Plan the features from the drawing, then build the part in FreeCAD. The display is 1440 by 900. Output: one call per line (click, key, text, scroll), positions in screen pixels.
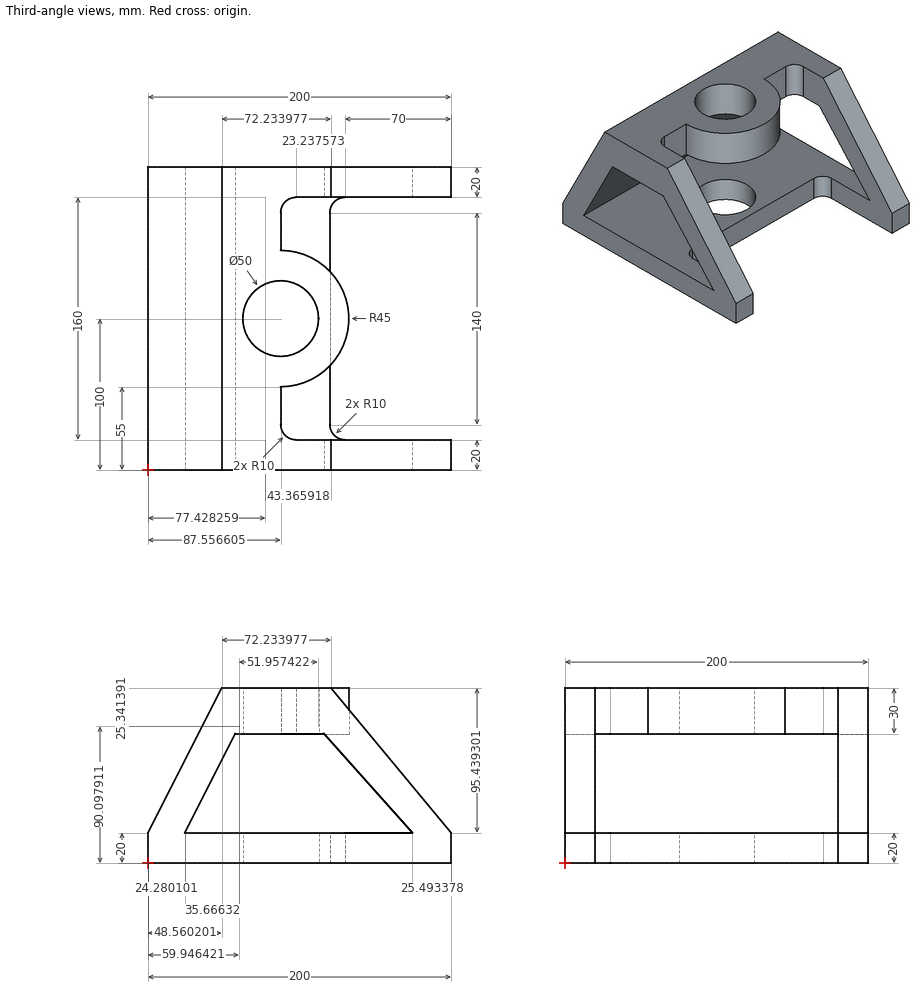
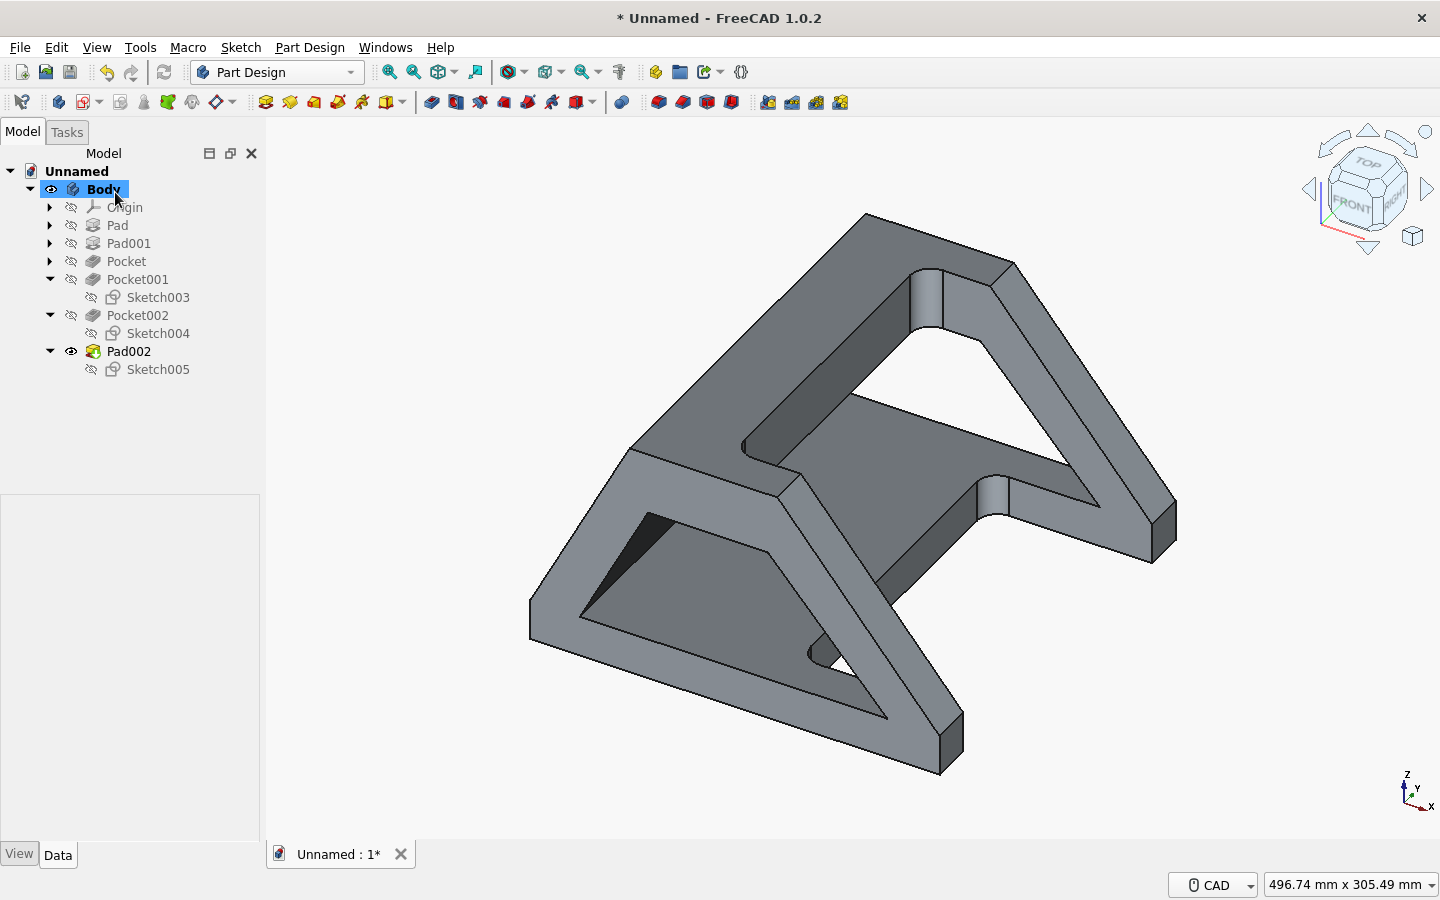
click(847, 273)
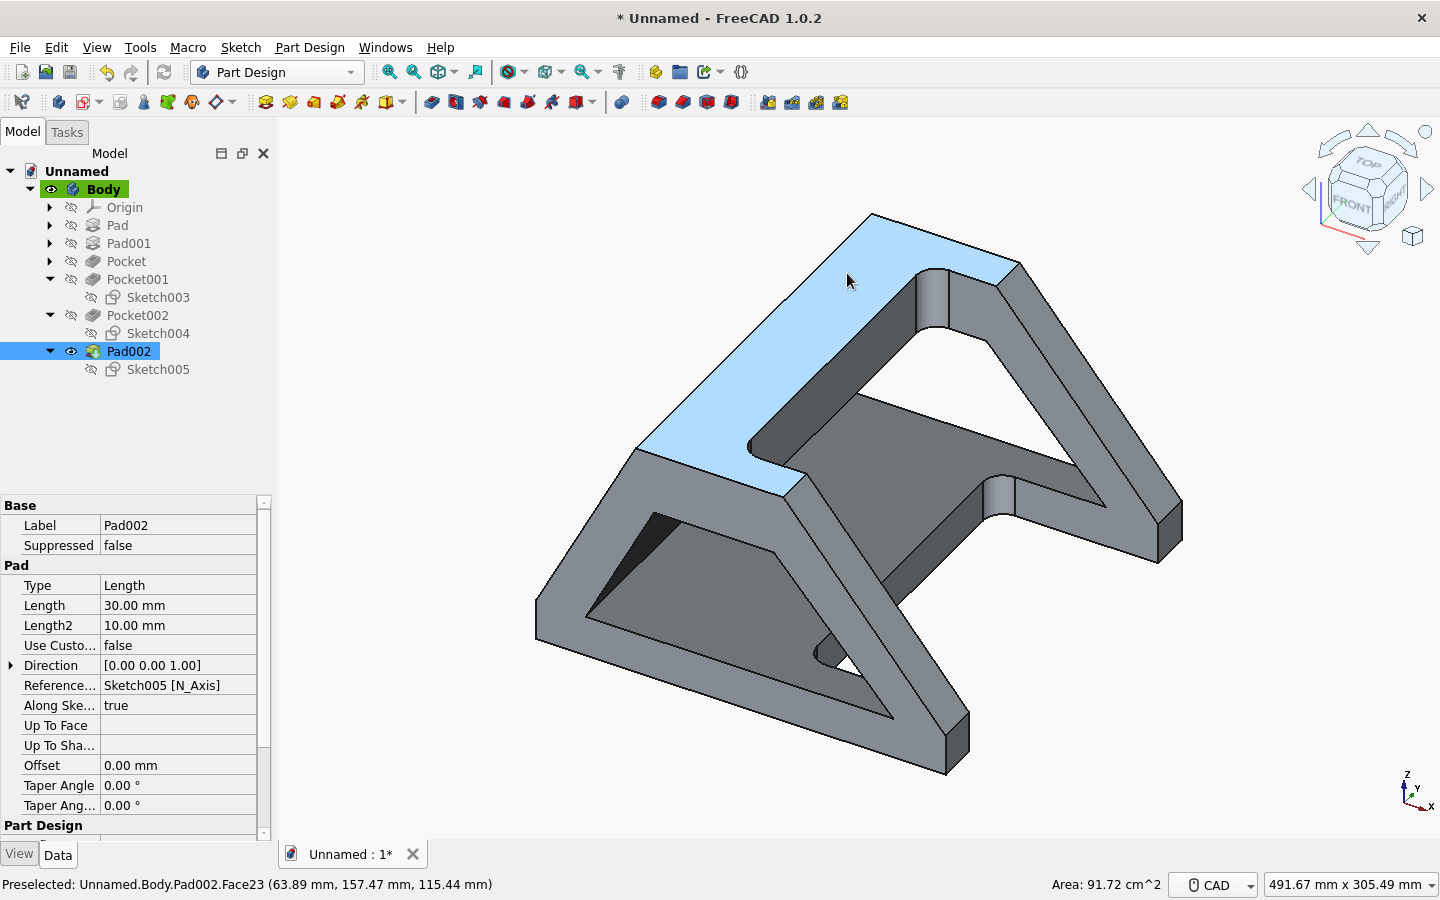
click(84, 102)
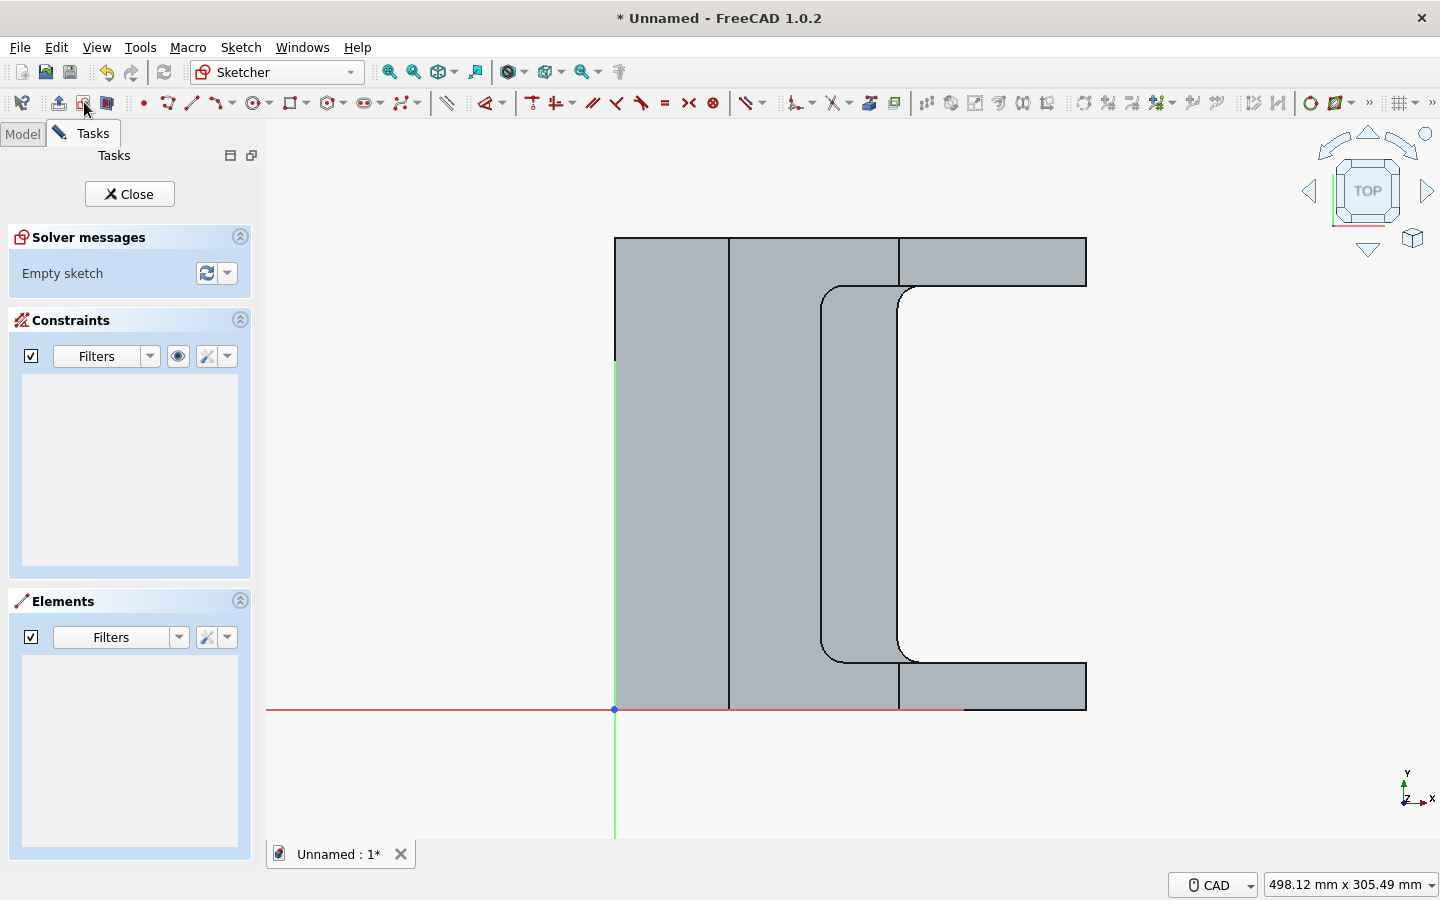
scroll(743, 661, up, 2)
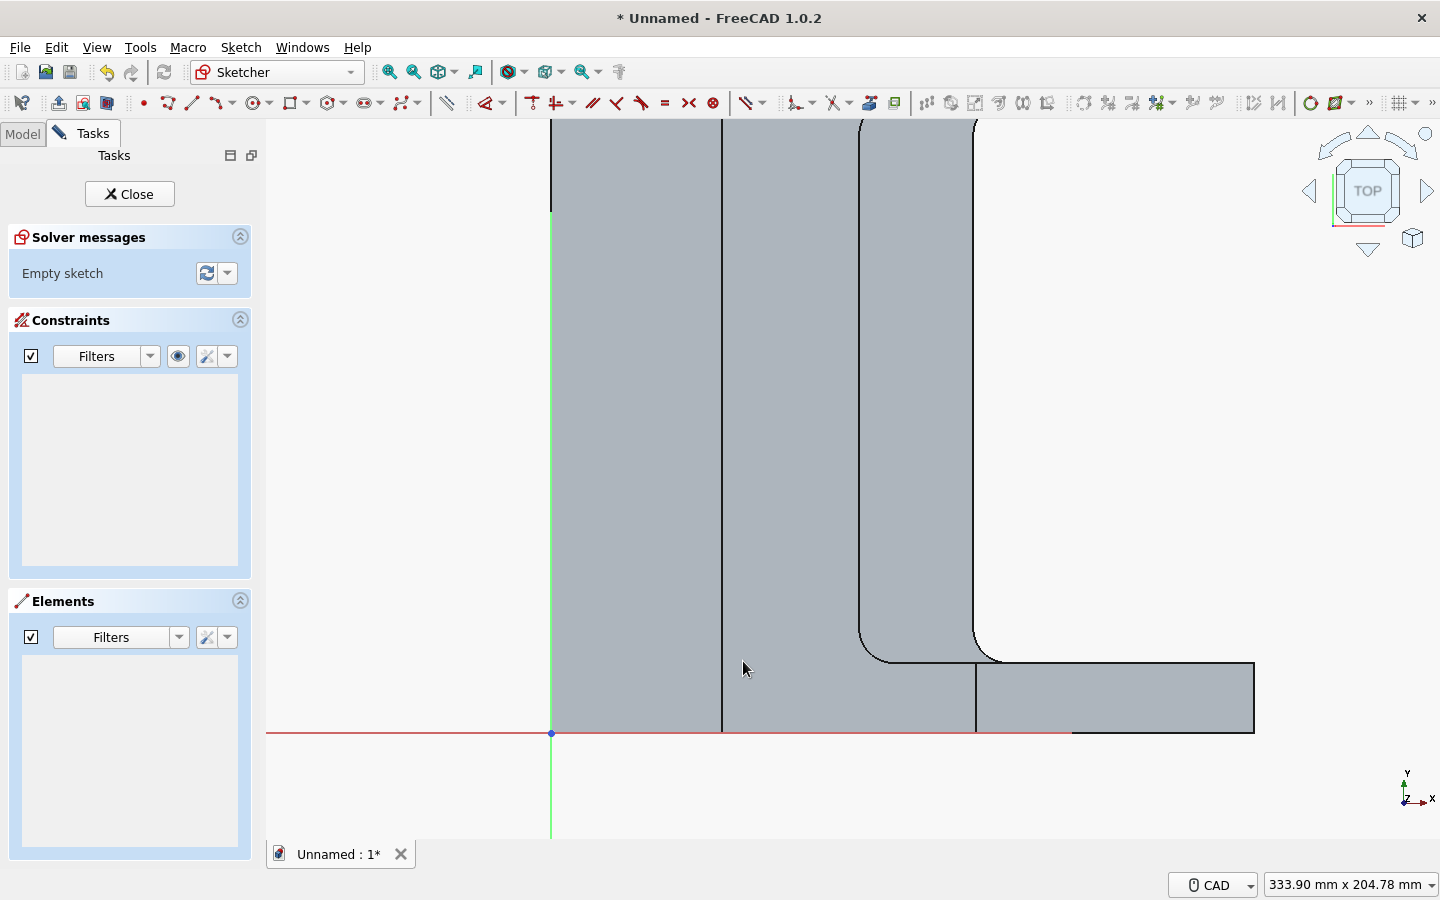
key(g)
key(l)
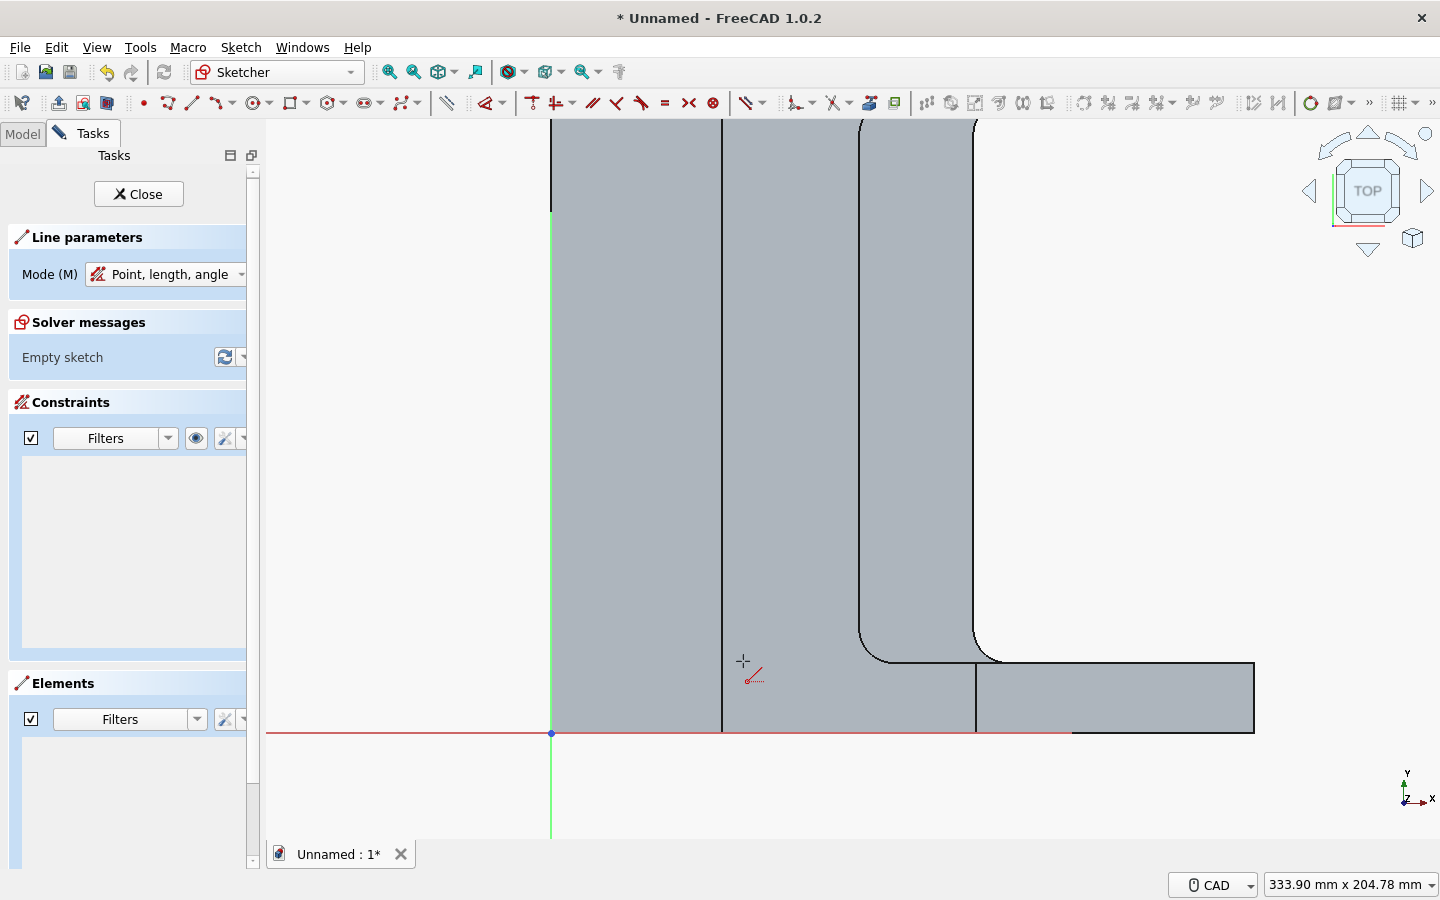
click(859, 224)
click(859, 540)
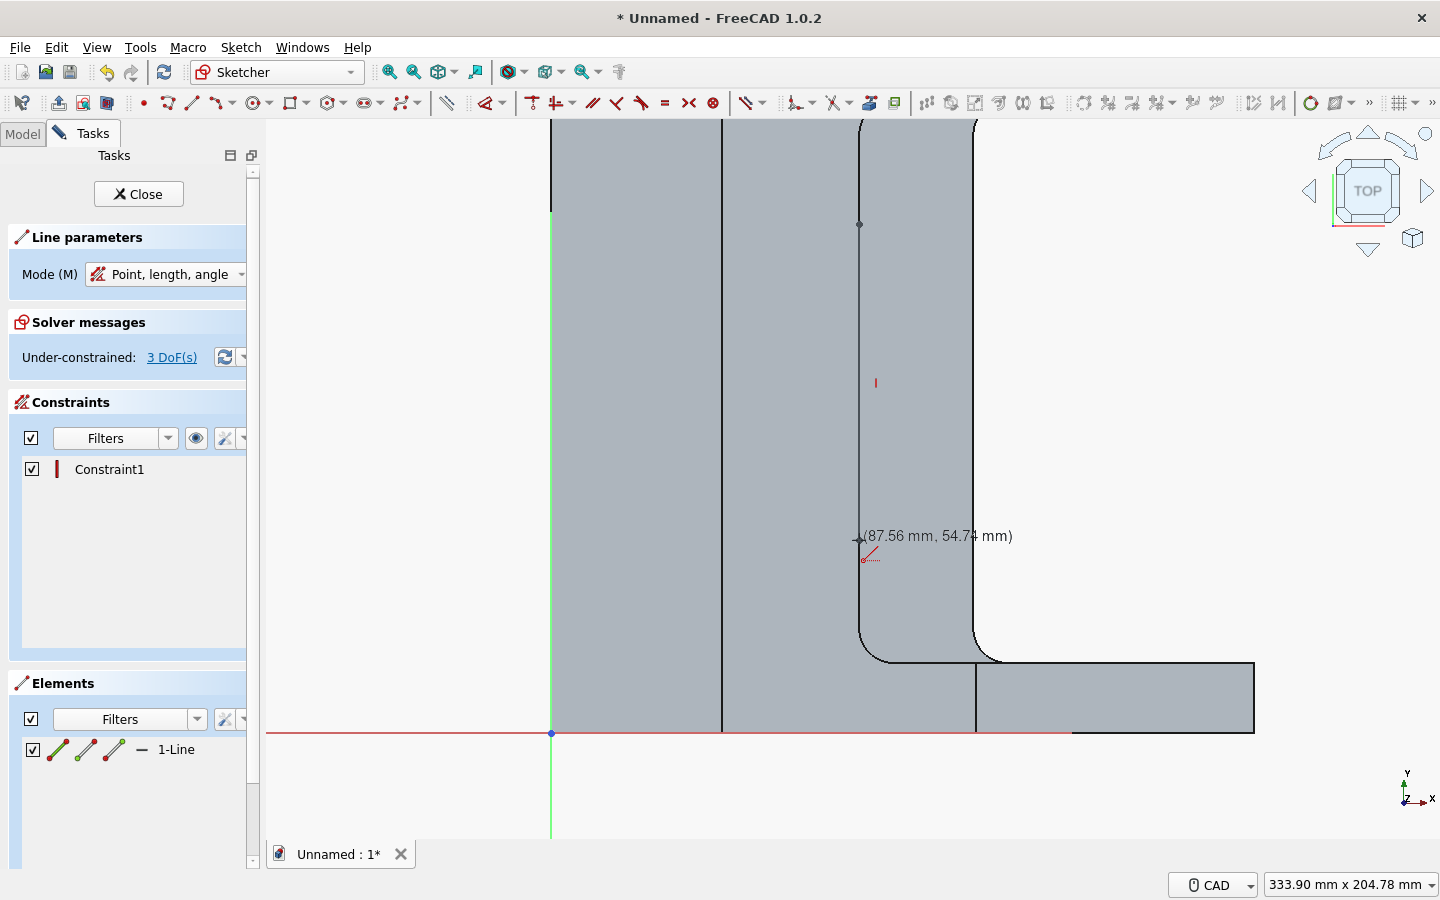
click(216, 104)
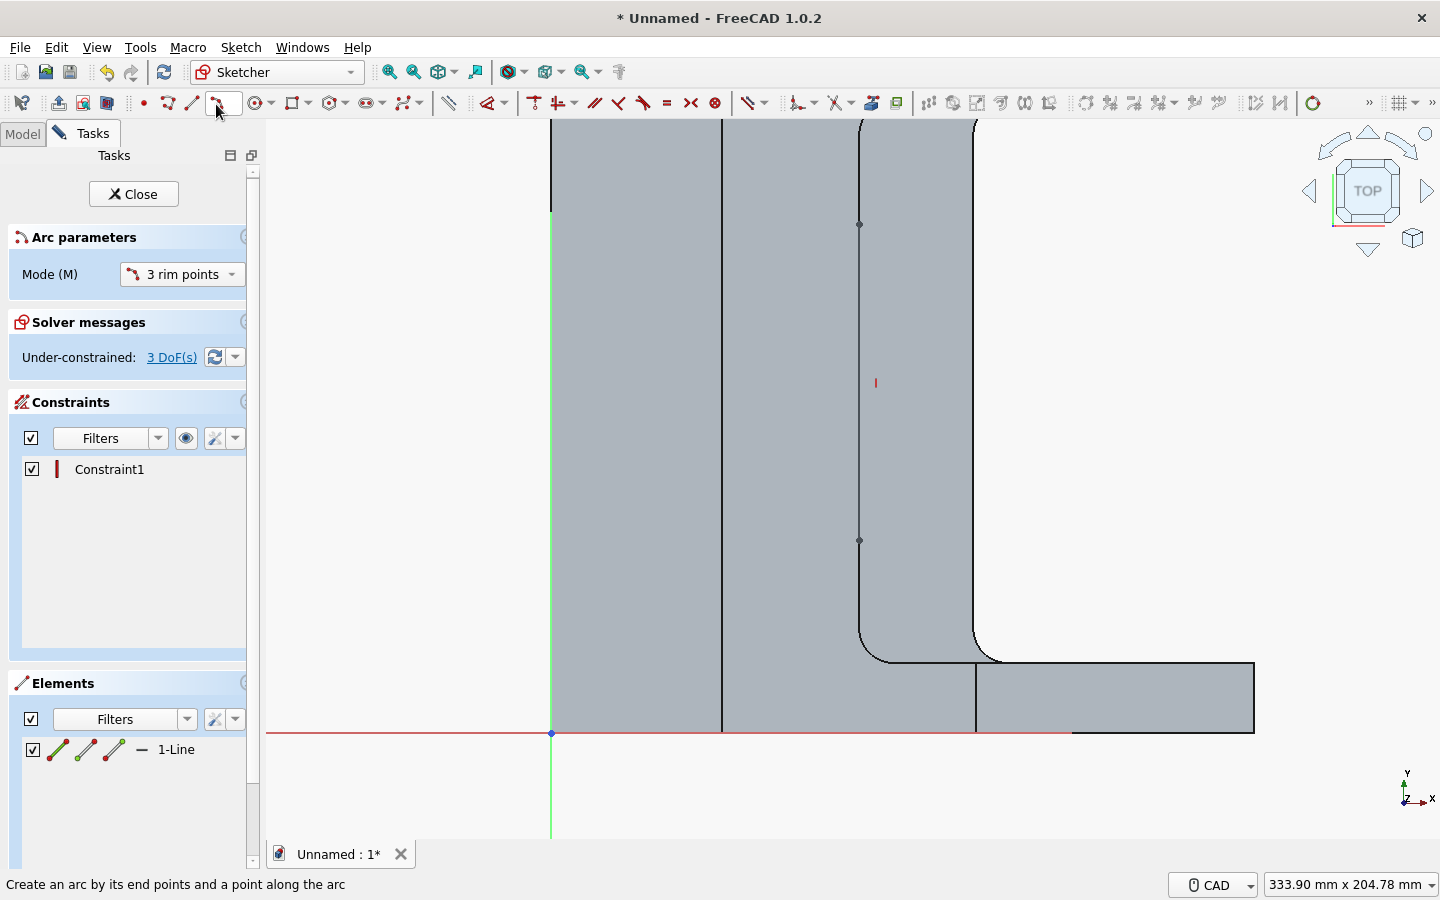
click(859, 541)
click(859, 225)
click(1017, 382)
key(Escape)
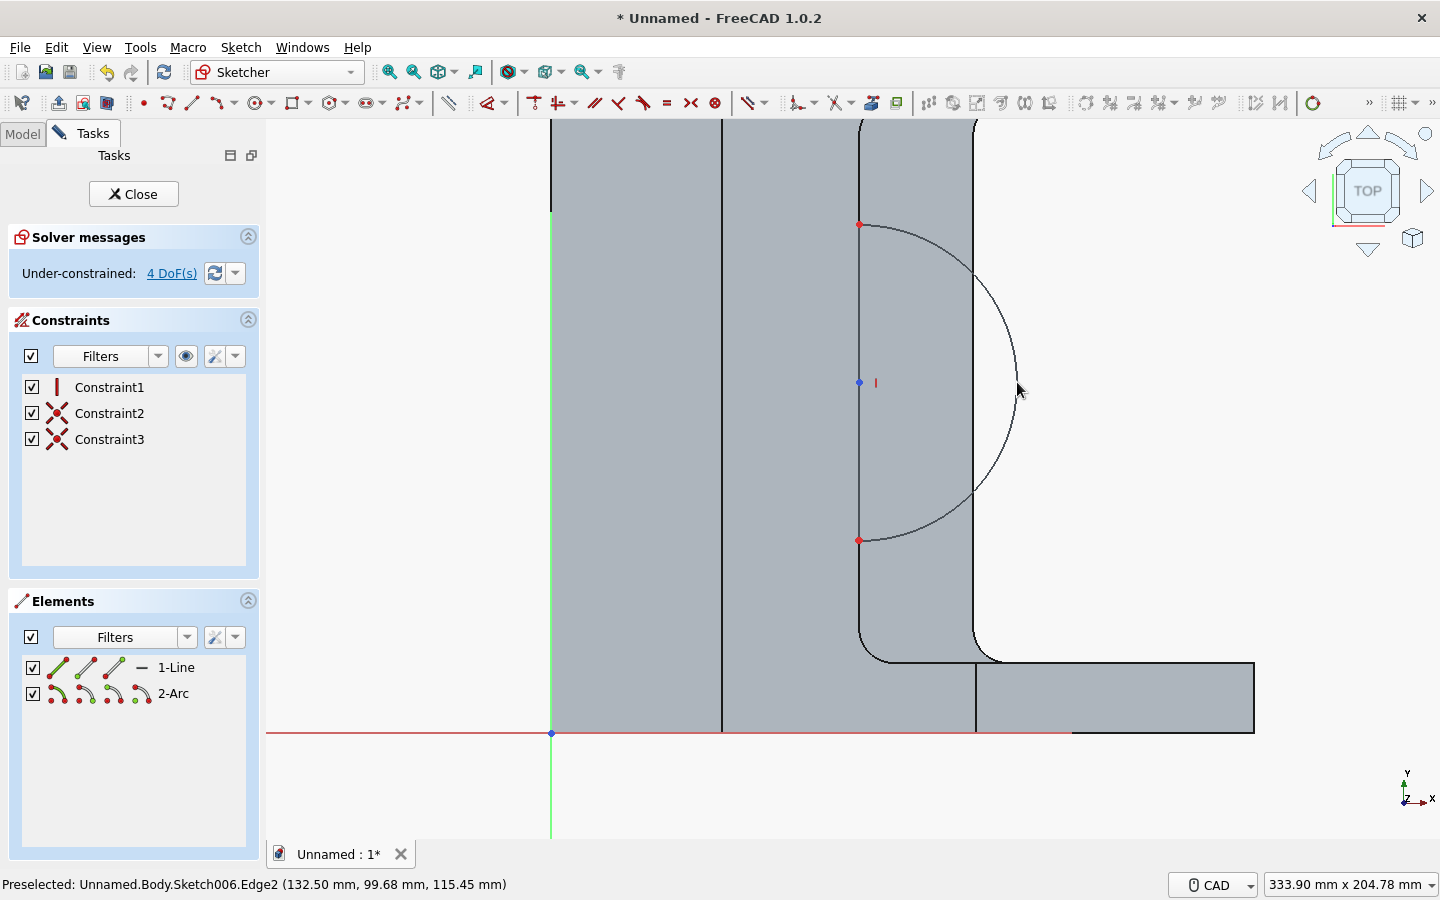
click(488, 104)